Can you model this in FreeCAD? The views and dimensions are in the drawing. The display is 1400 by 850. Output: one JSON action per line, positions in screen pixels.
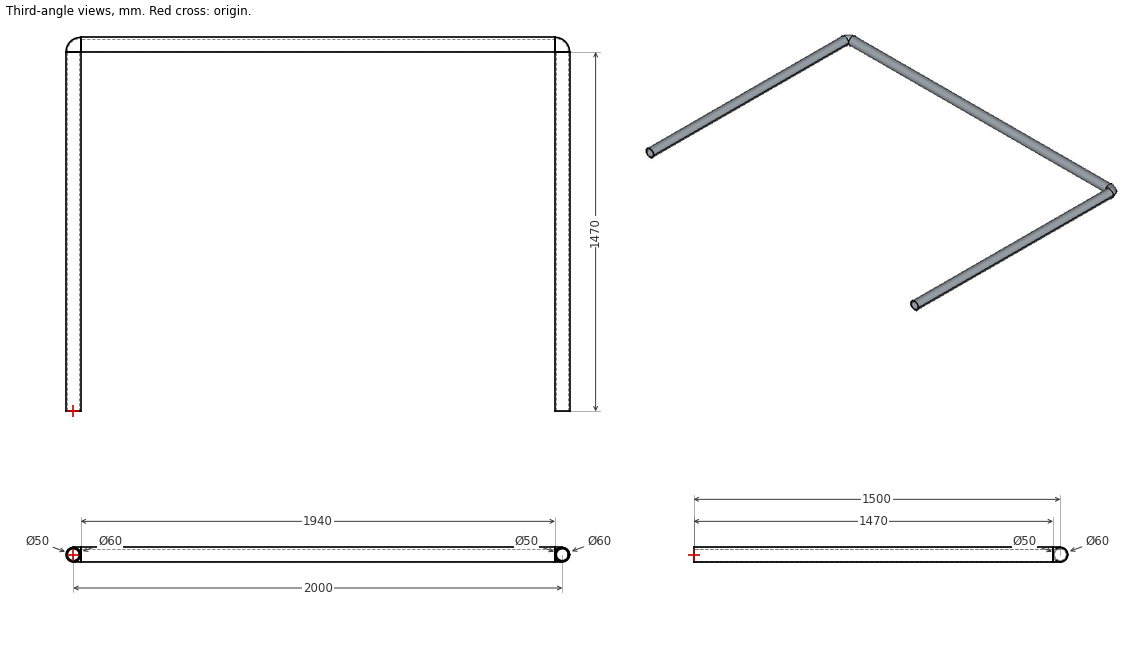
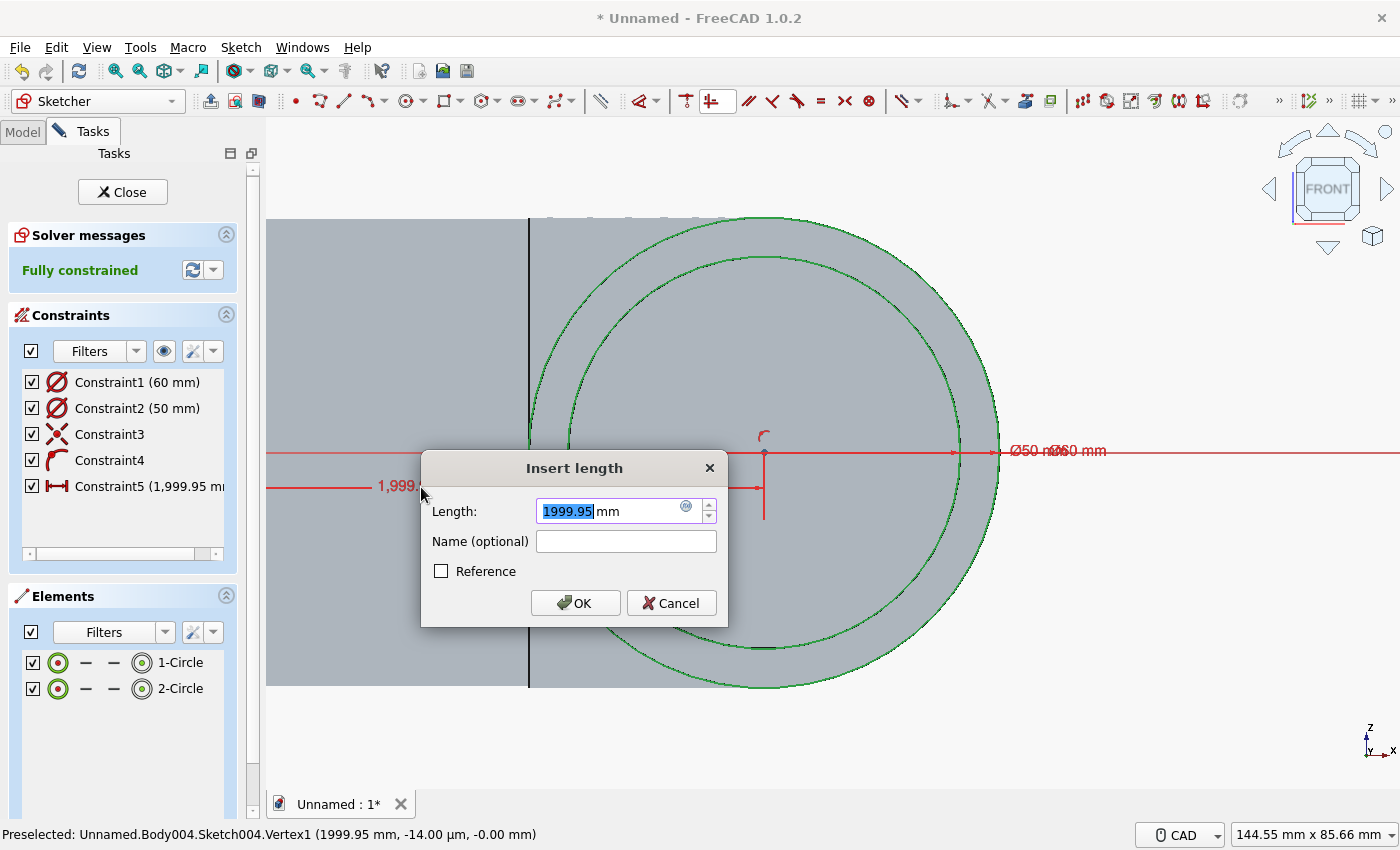
{"action": "type", "text": "2000"}
{"action": "key", "text": "Return"}
{"action": "key", "text": "Escape"}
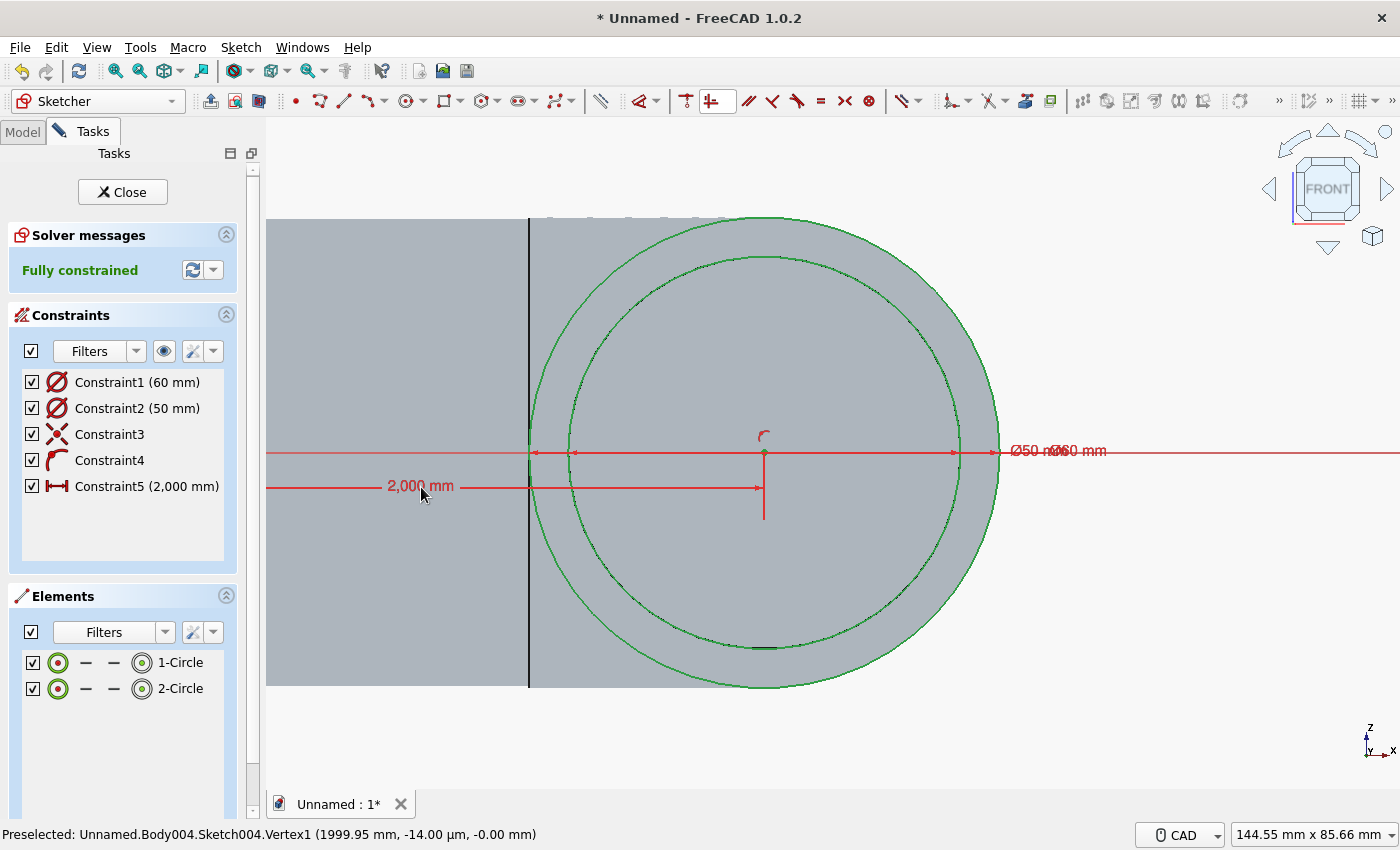
{"action": "left_click", "coordinate": [123, 192]}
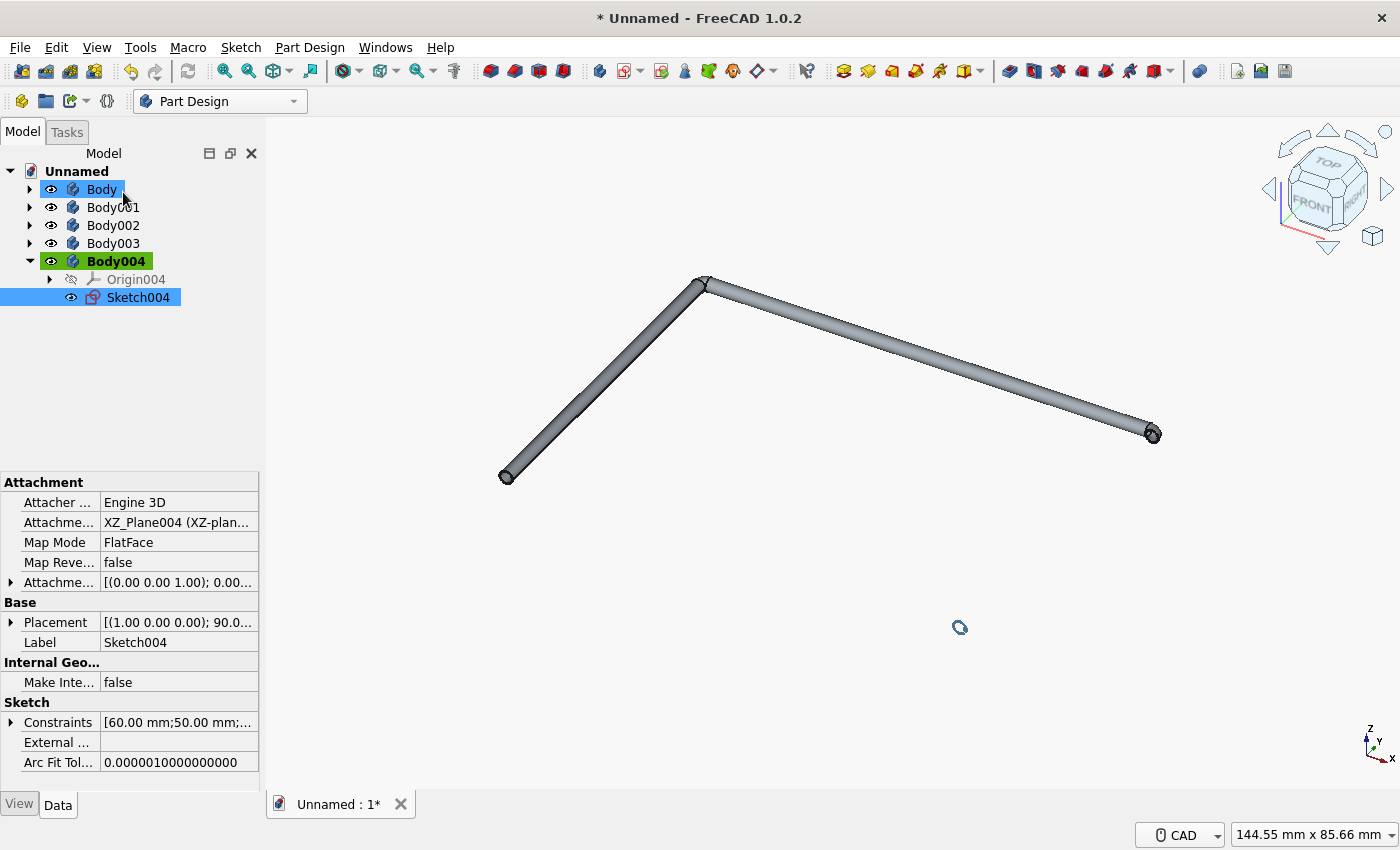
{"action": "left_click", "coordinate": [844, 72]}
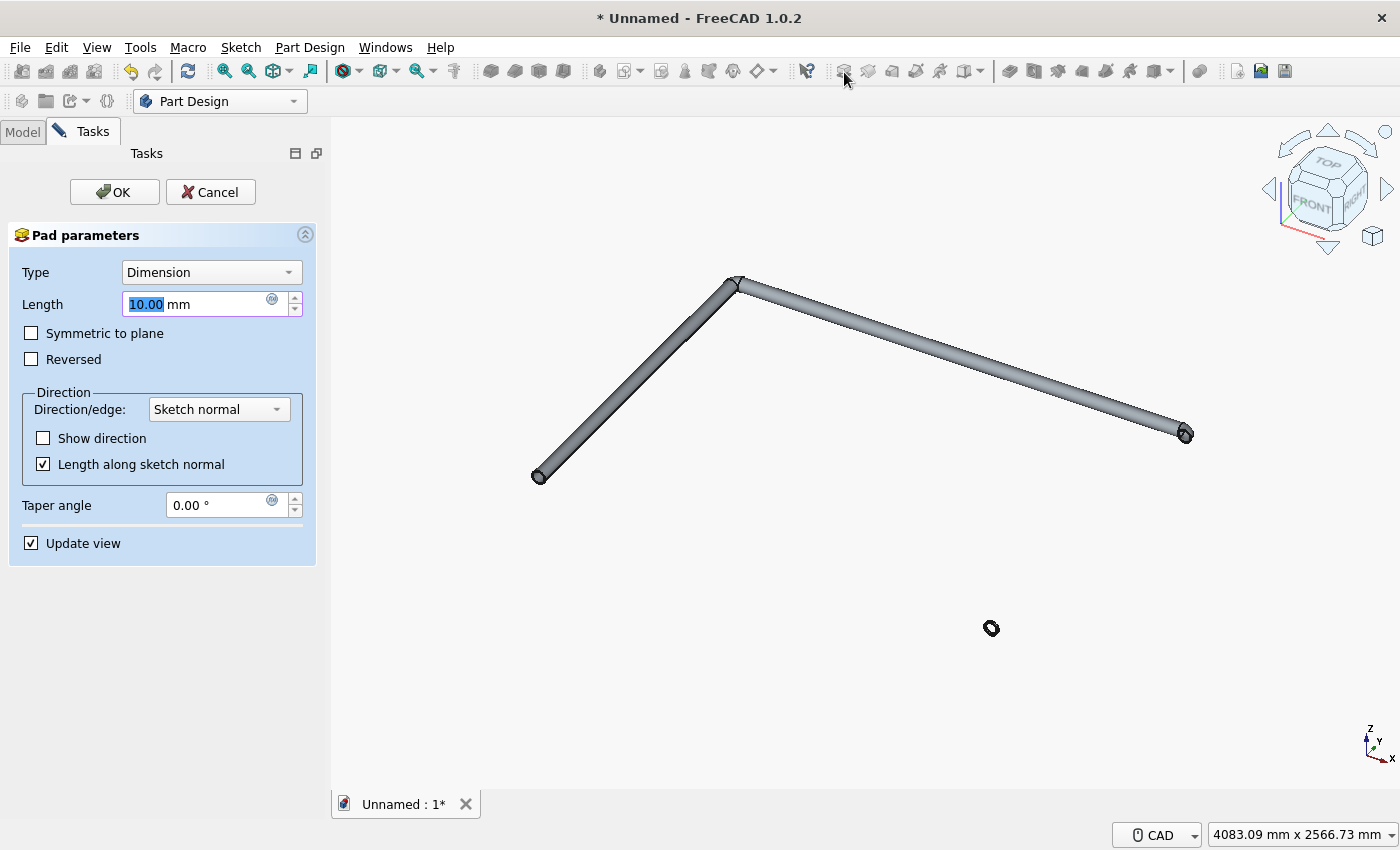
{"action": "type", "text": "1470"}
{"action": "key", "text": "Tab"}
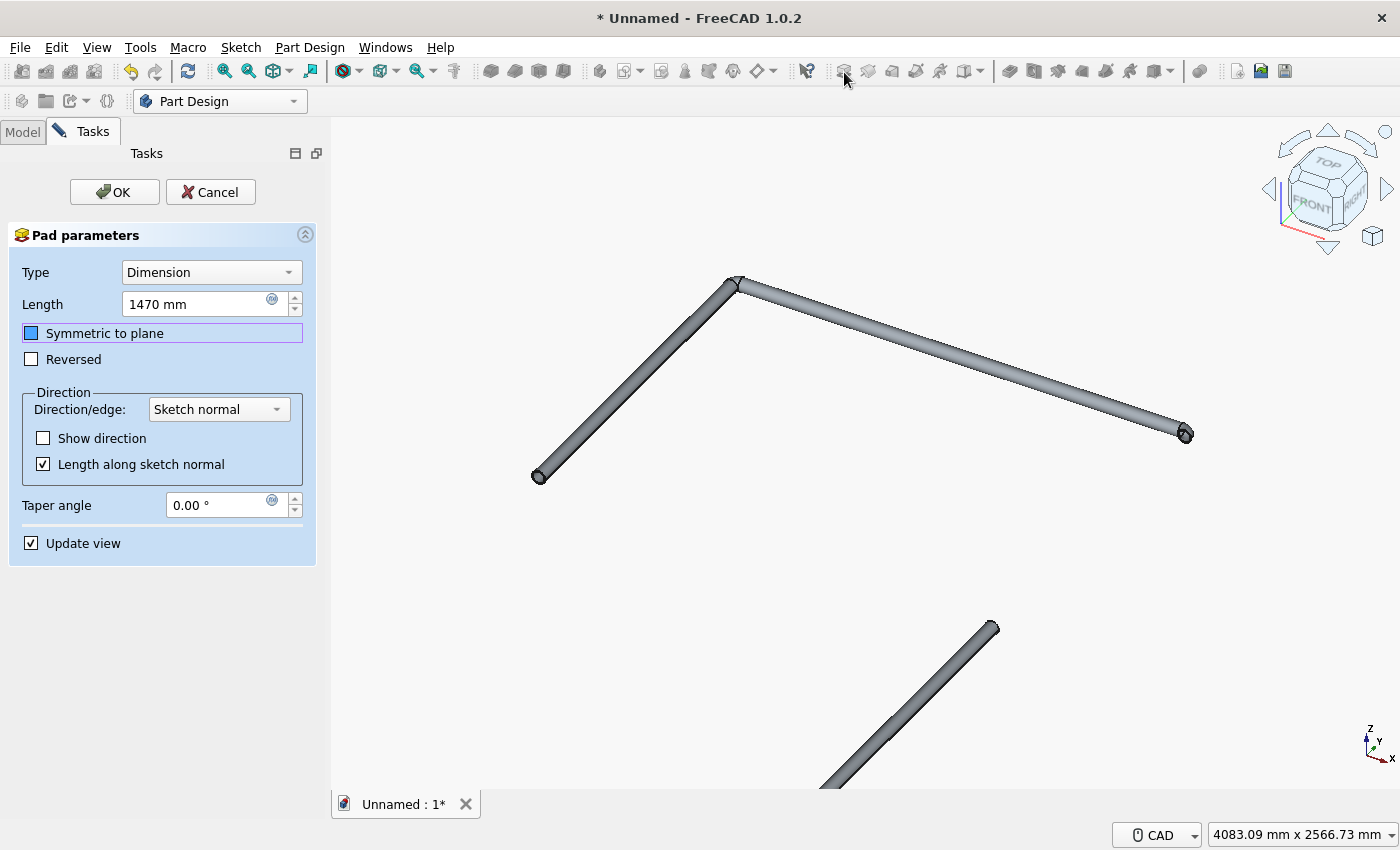
{"action": "left_click", "coordinate": [30, 359]}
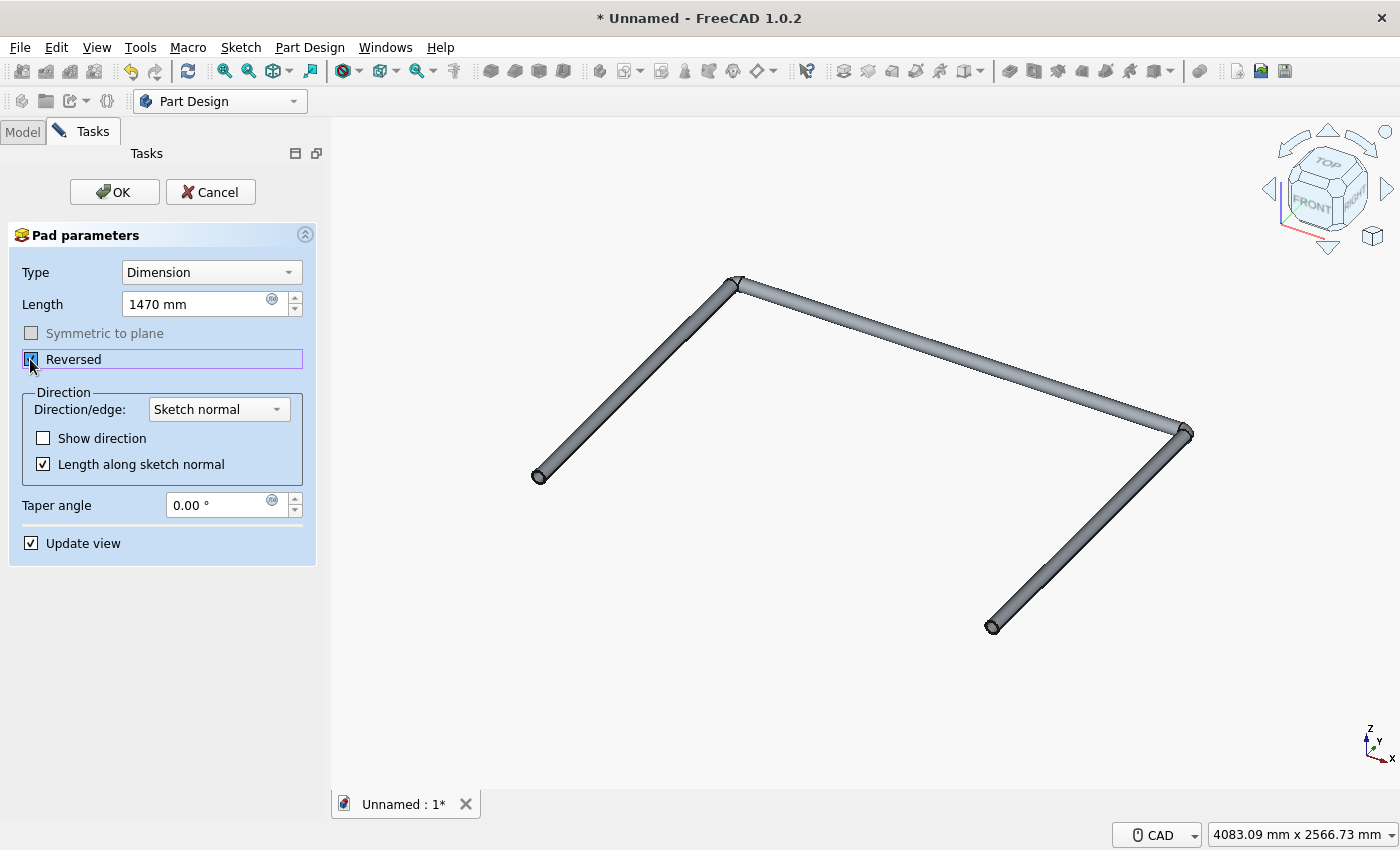
{"action": "left_click", "coordinate": [115, 192]}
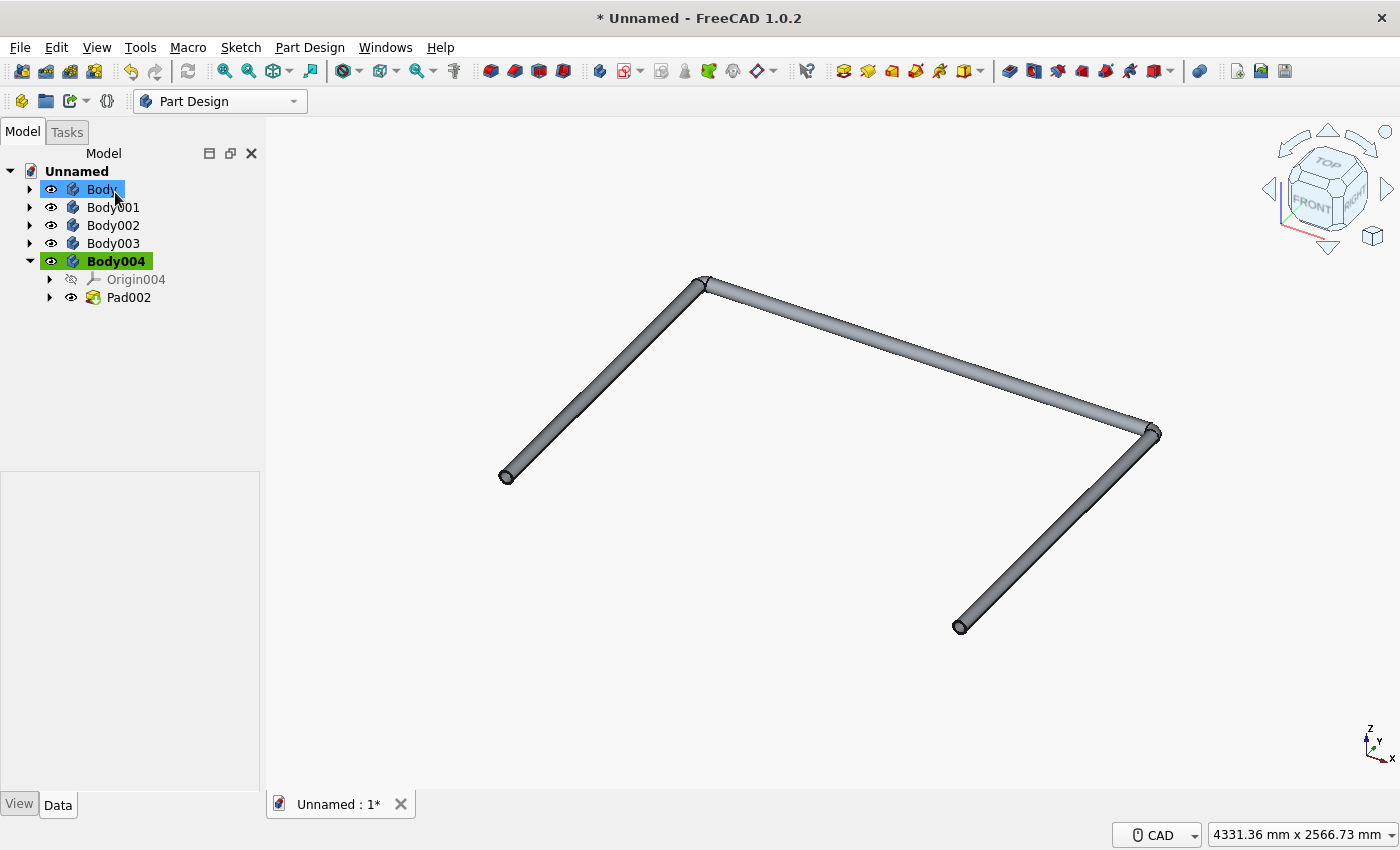
{"action": "key", "text": "0"}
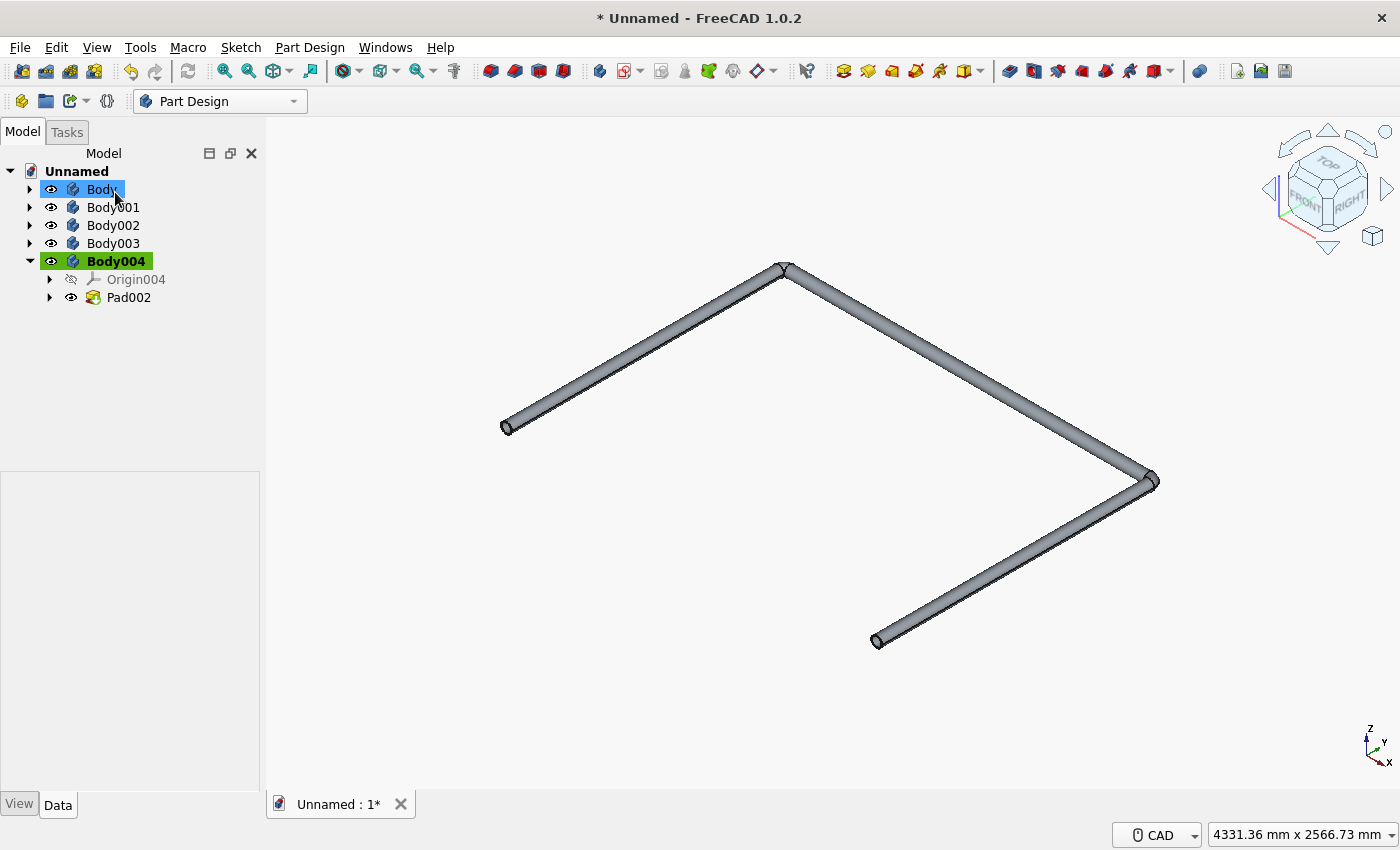
{"action": "left_click", "coordinate": [226, 72]}